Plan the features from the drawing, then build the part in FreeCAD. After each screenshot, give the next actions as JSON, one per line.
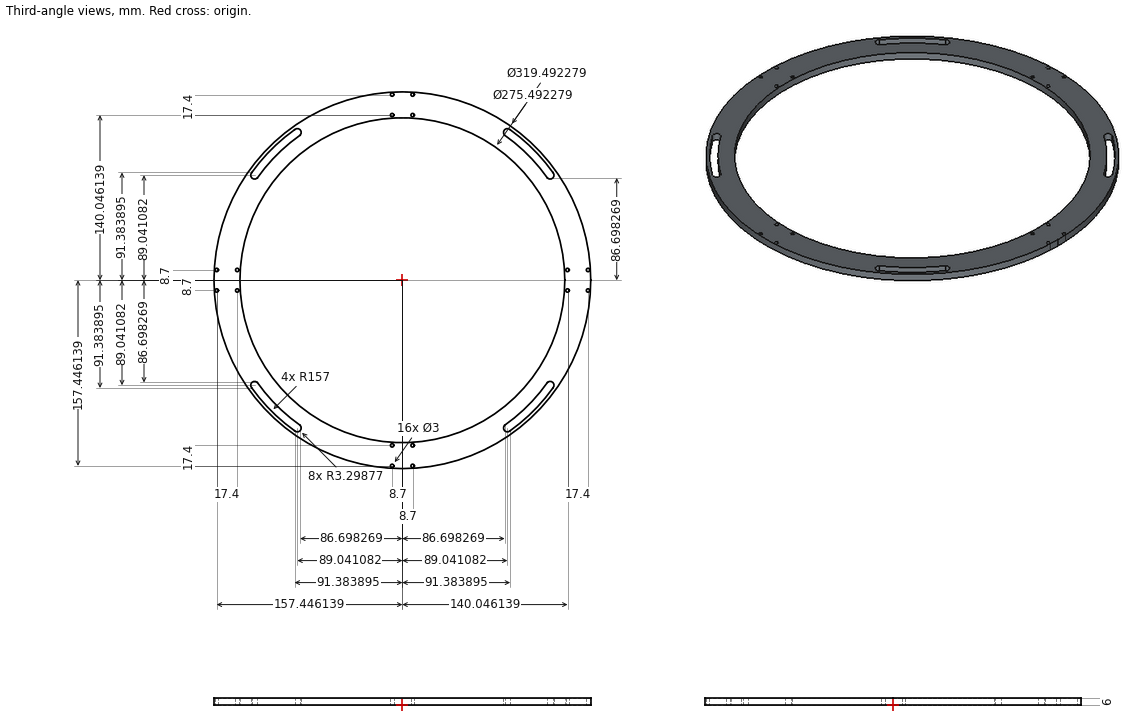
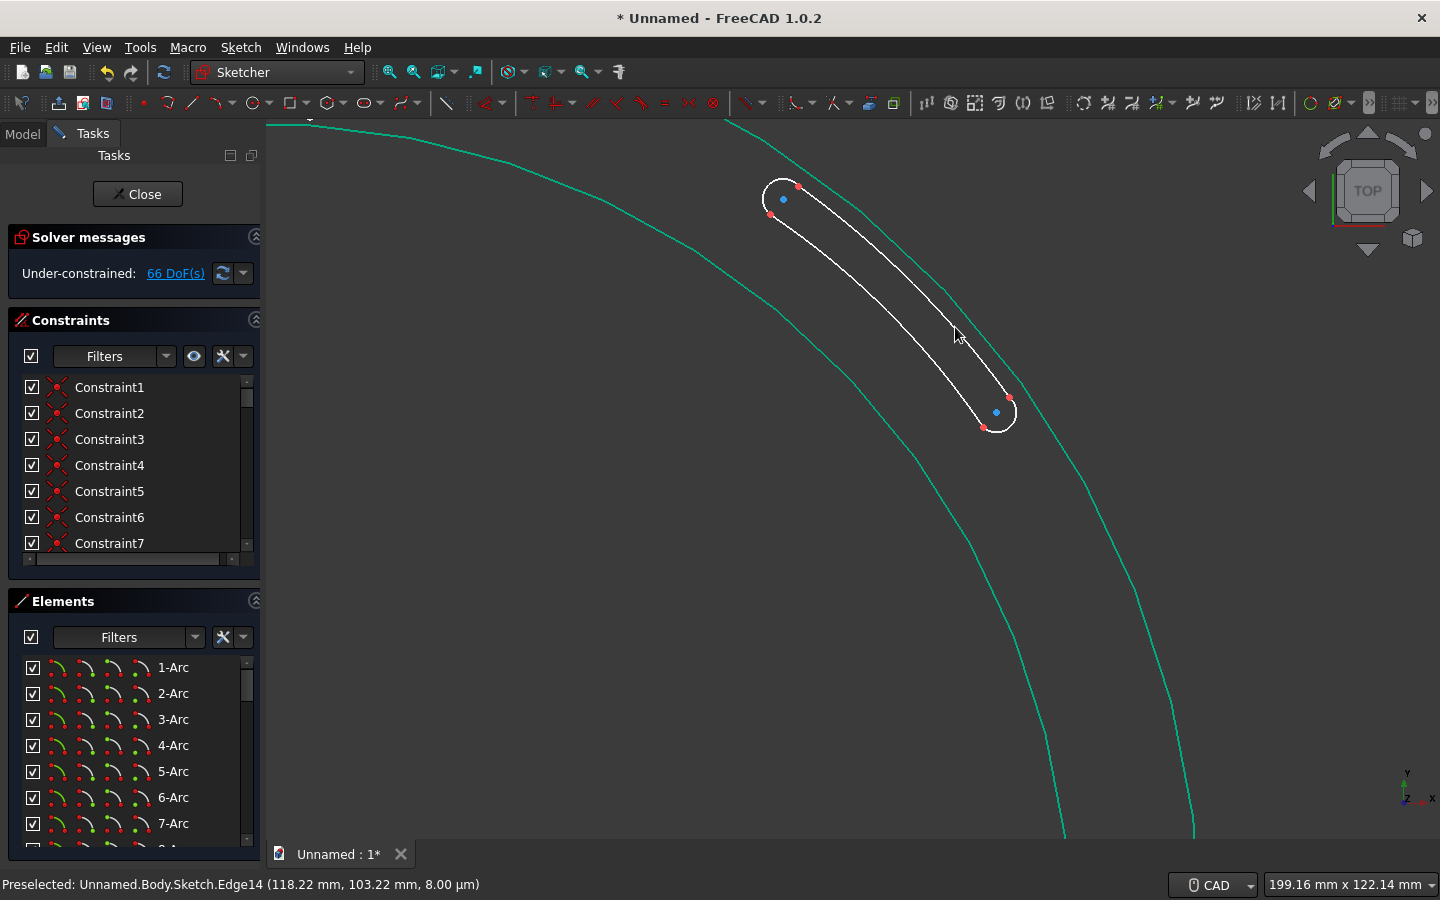
{"action": "left_click", "coordinate": [923, 268]}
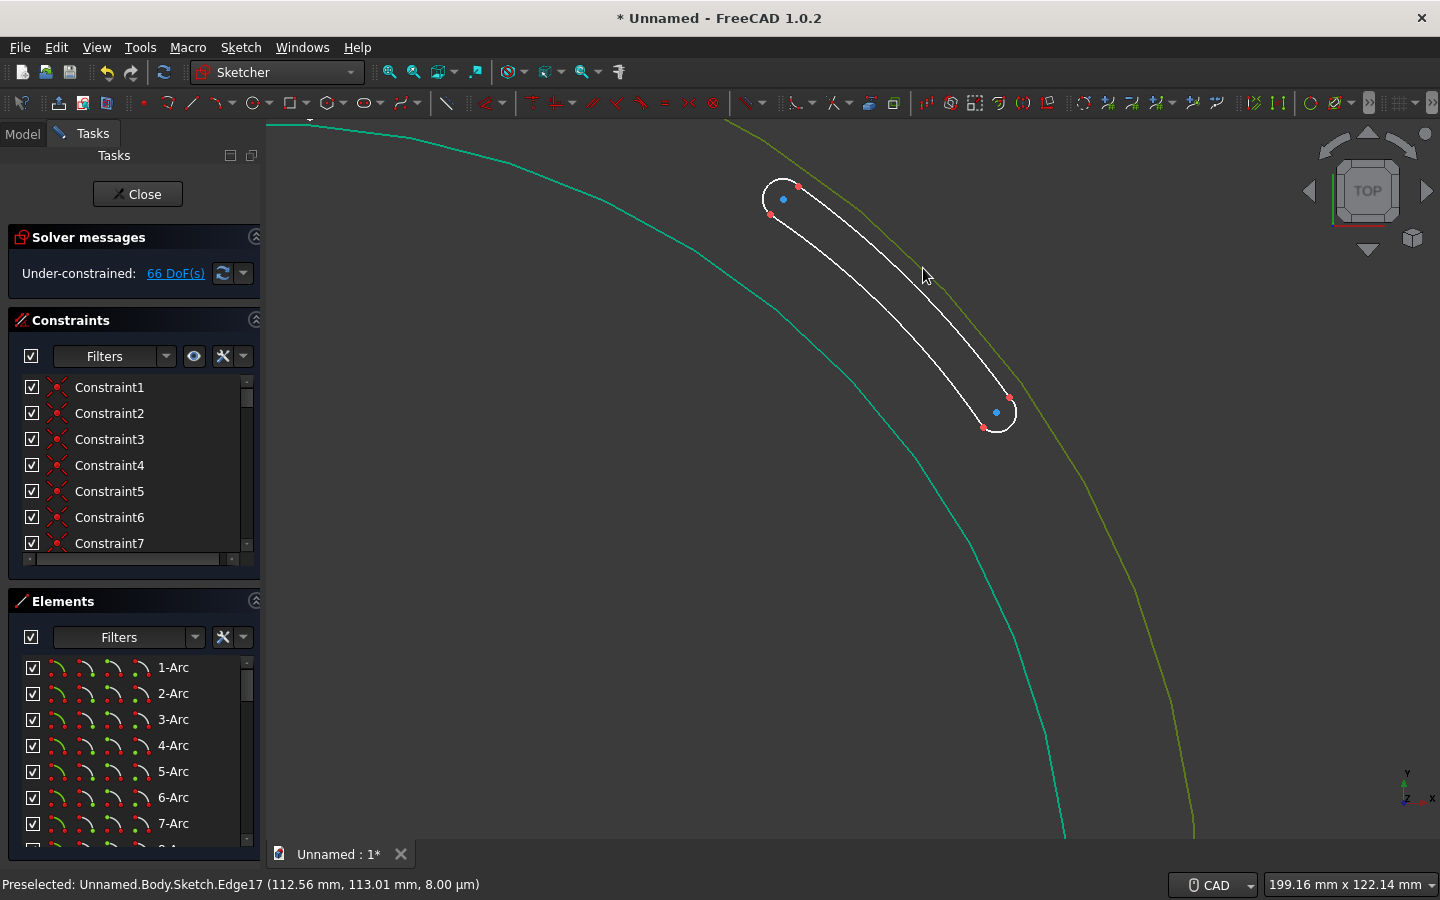
{"action": "left_click", "coordinate": [929, 355]}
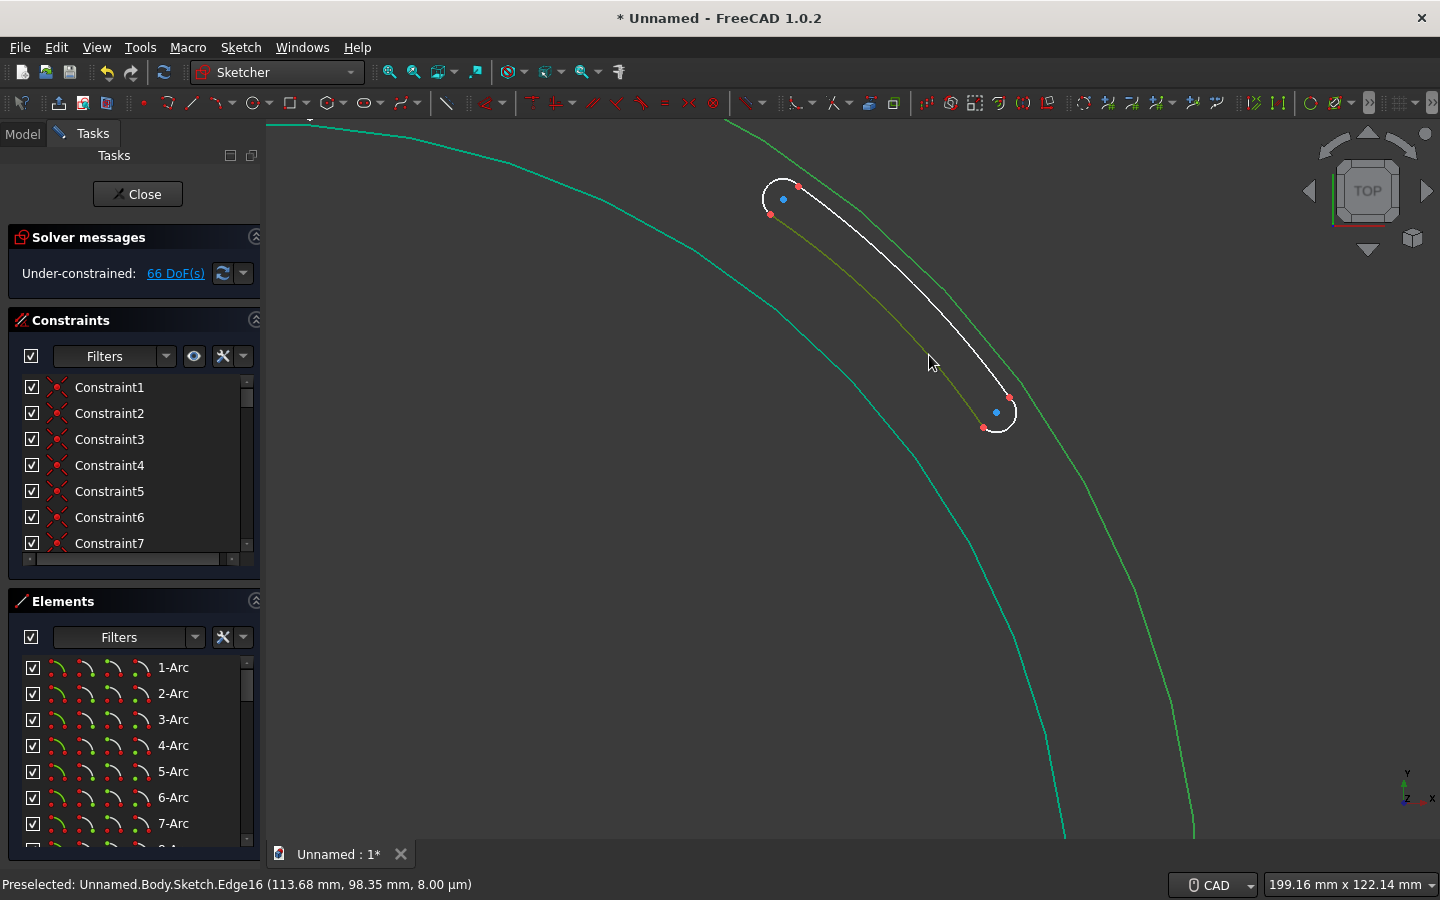
{"action": "key", "text": "c"}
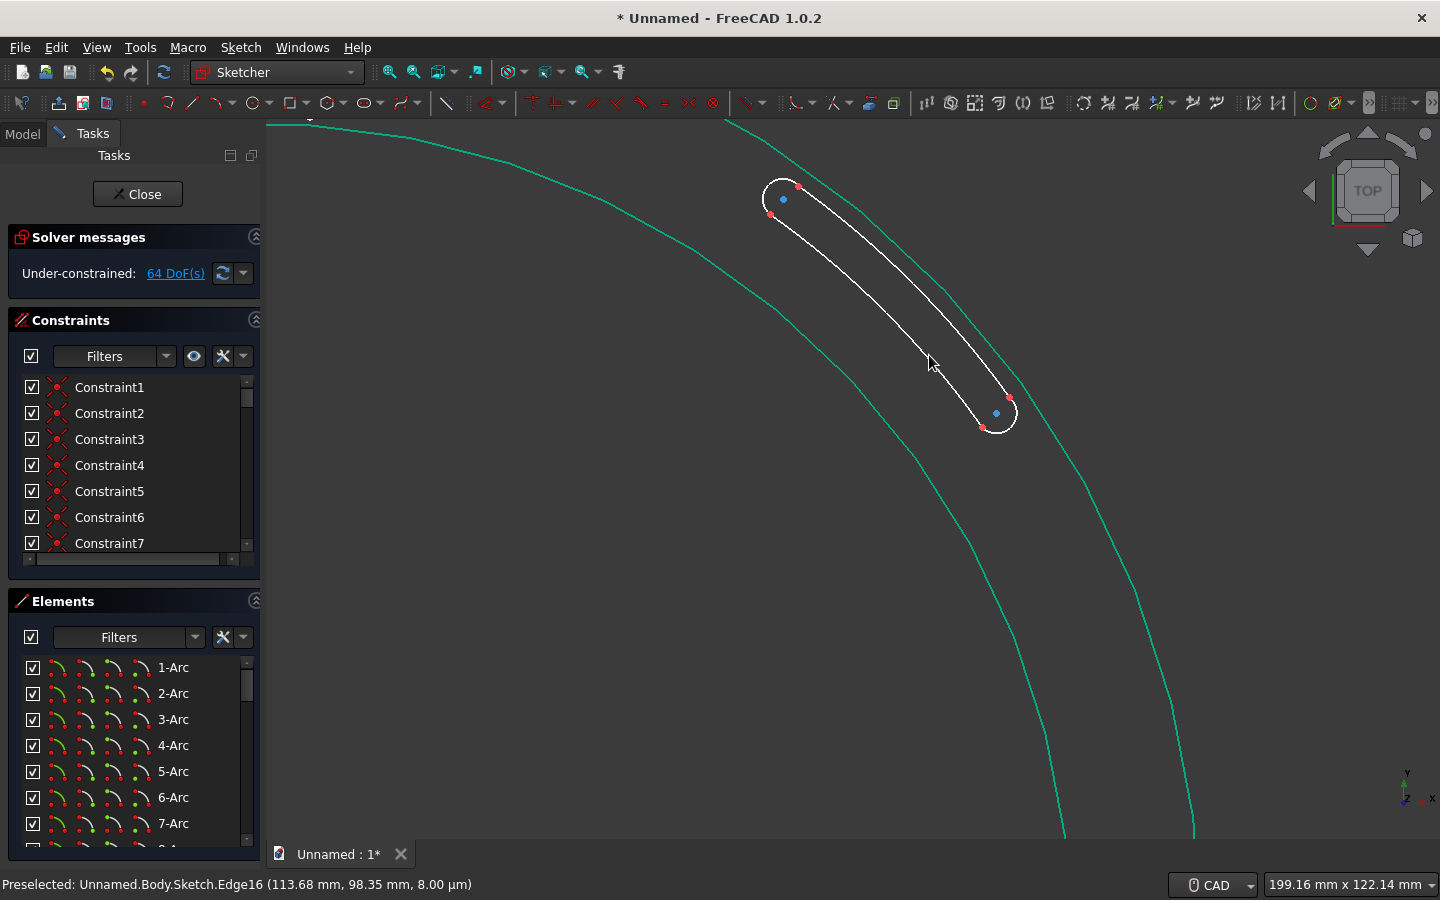
{"action": "scroll", "coordinate": [957, 329], "scroll_direction": "down", "scroll_amount": 7}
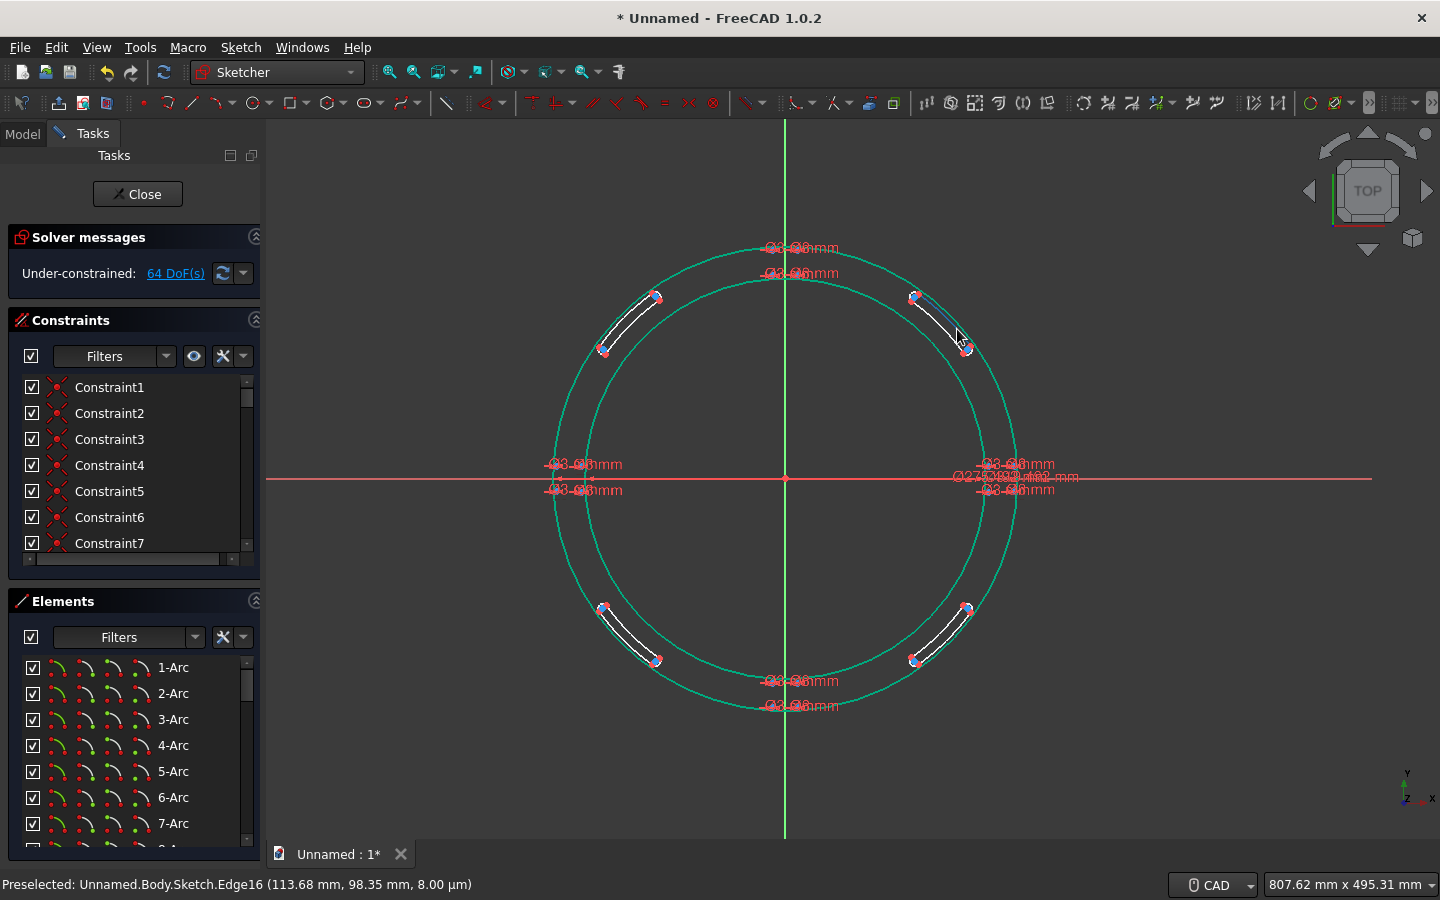
{"action": "scroll", "coordinate": [657, 666], "scroll_direction": "up", "scroll_amount": 7}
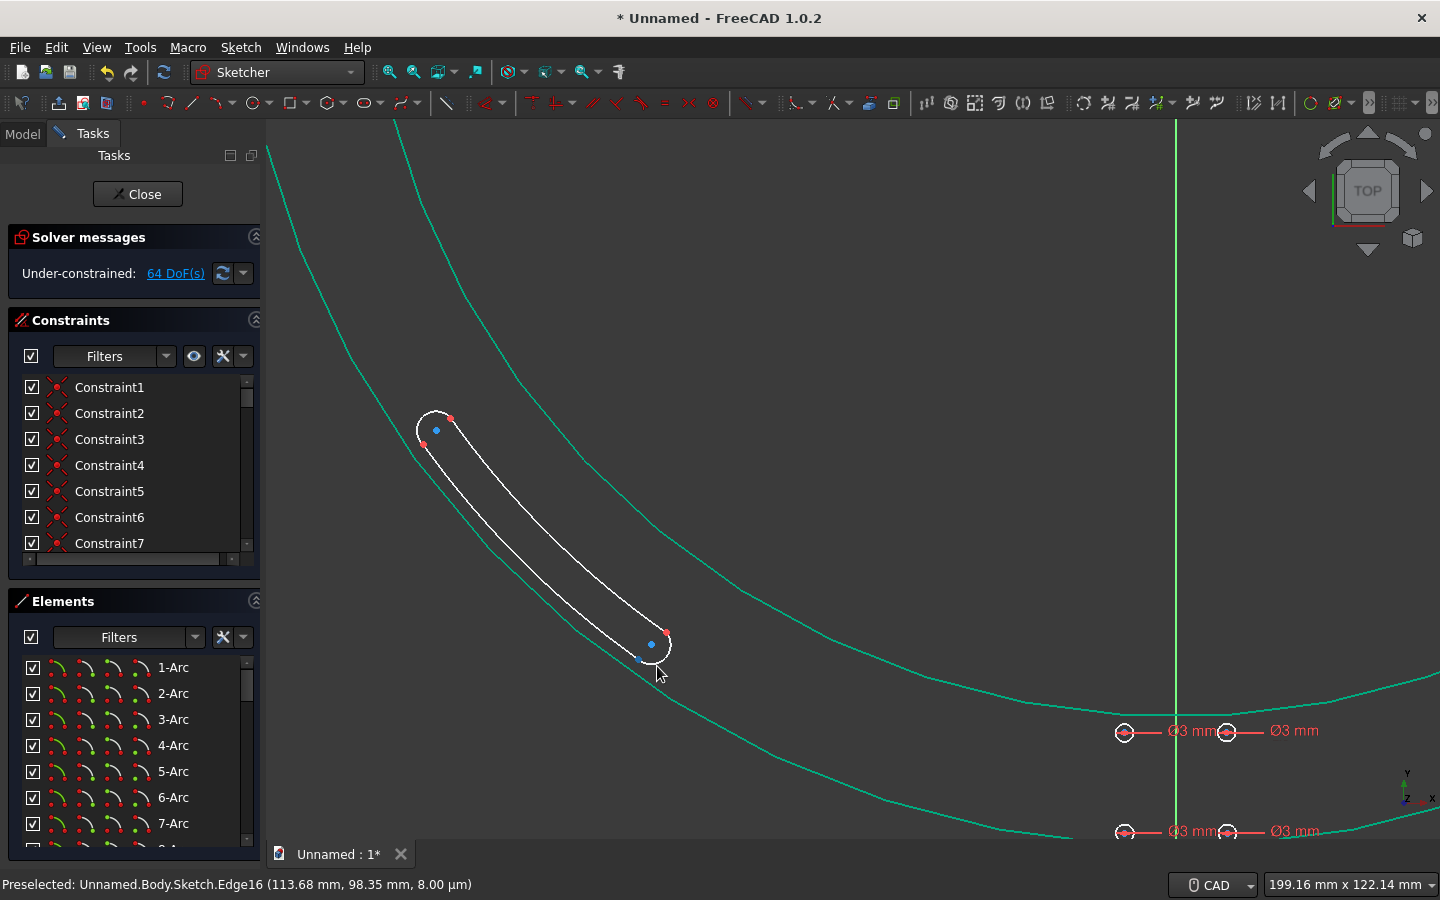
{"action": "left_click", "coordinate": [654, 664]}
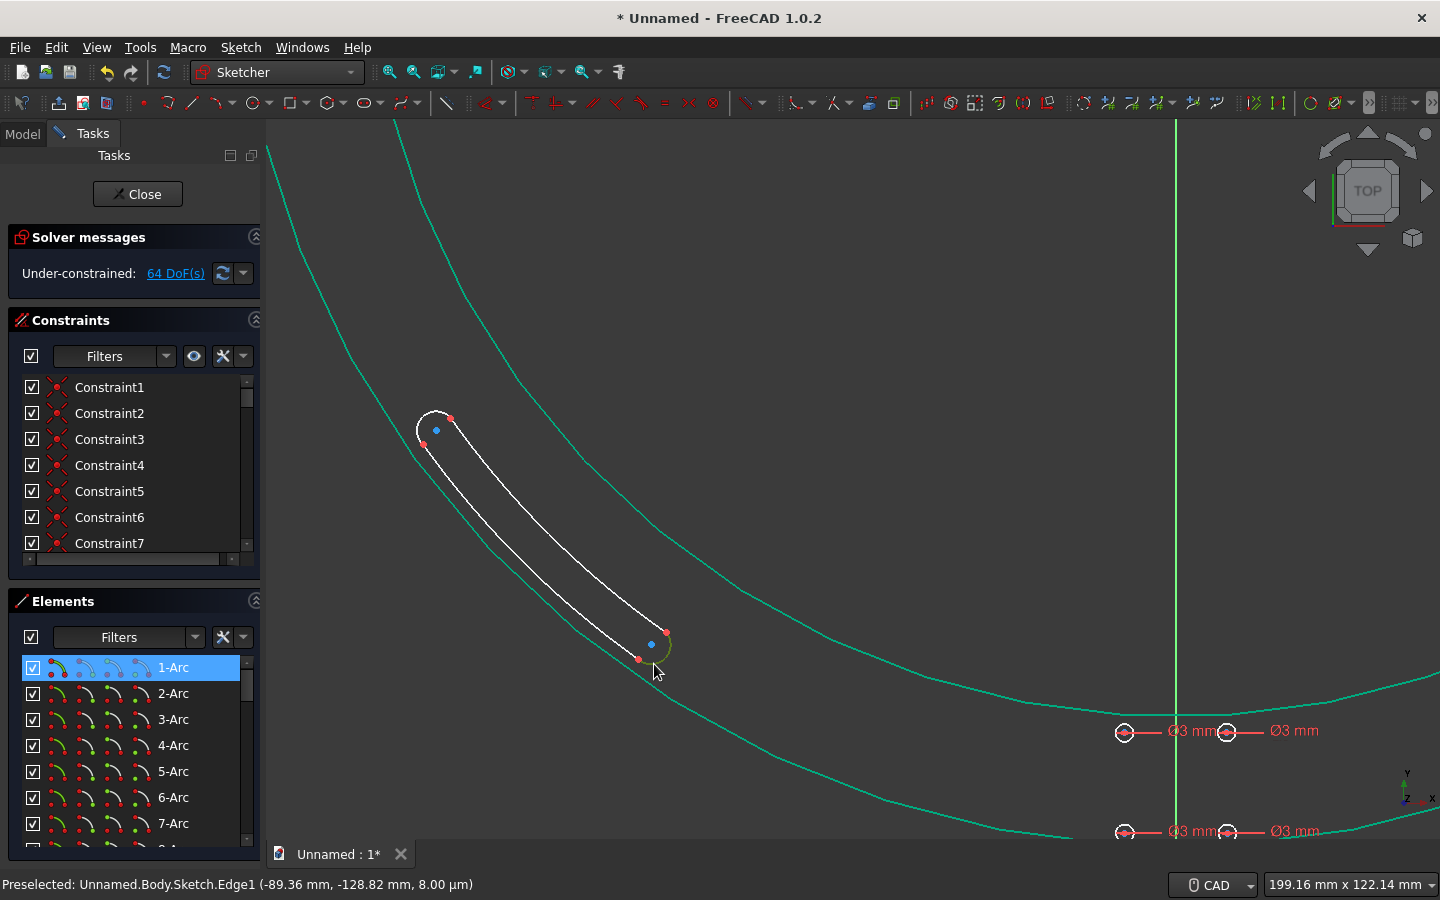
{"action": "scroll", "coordinate": [656, 667], "scroll_direction": "down", "scroll_amount": 7}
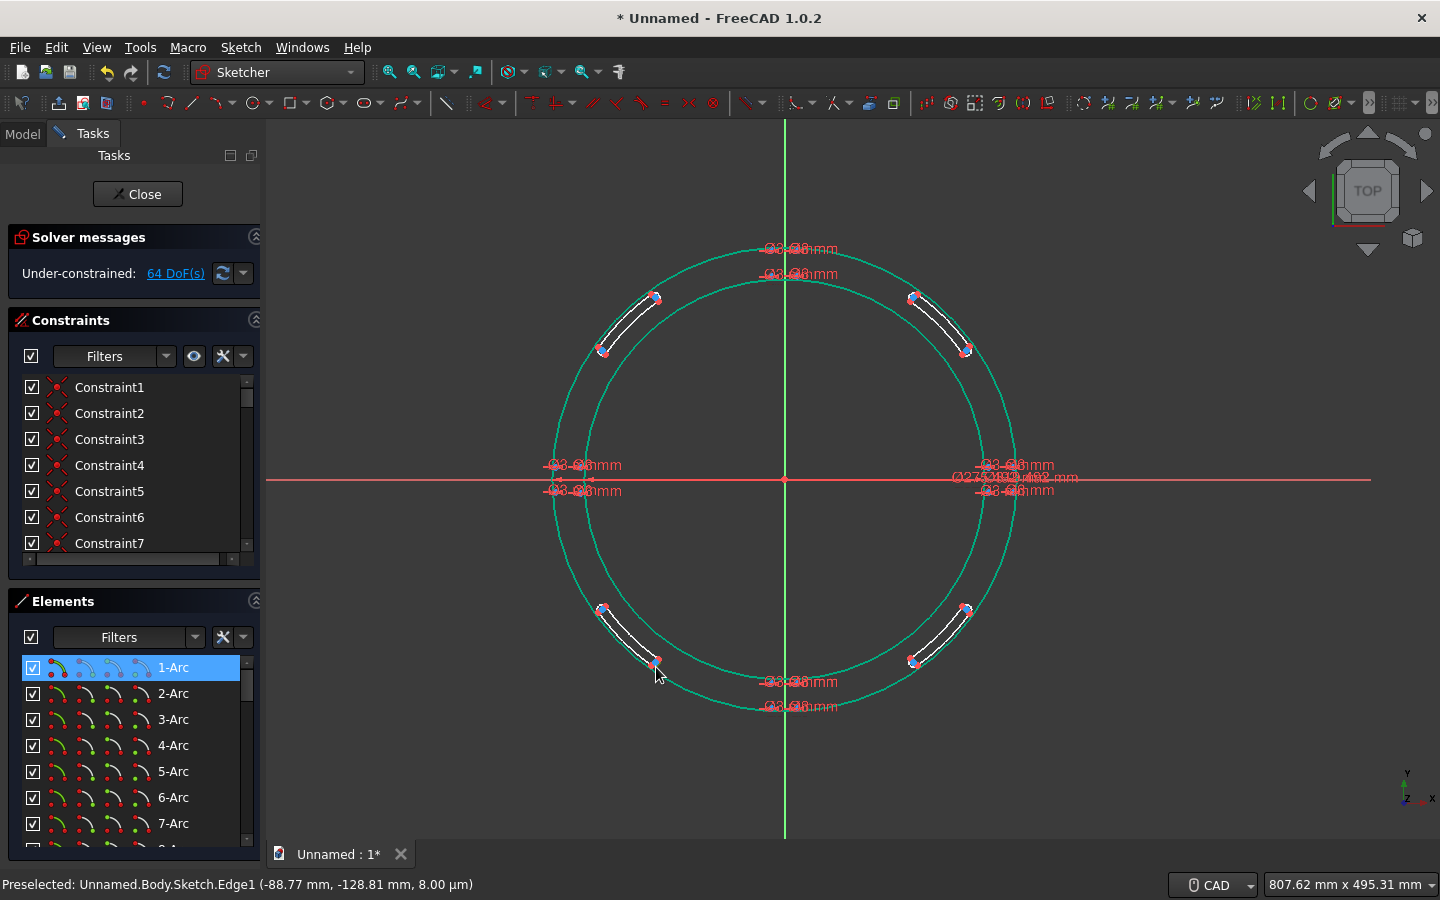
{"action": "scroll", "coordinate": [971, 609], "scroll_direction": "up", "scroll_amount": 6}